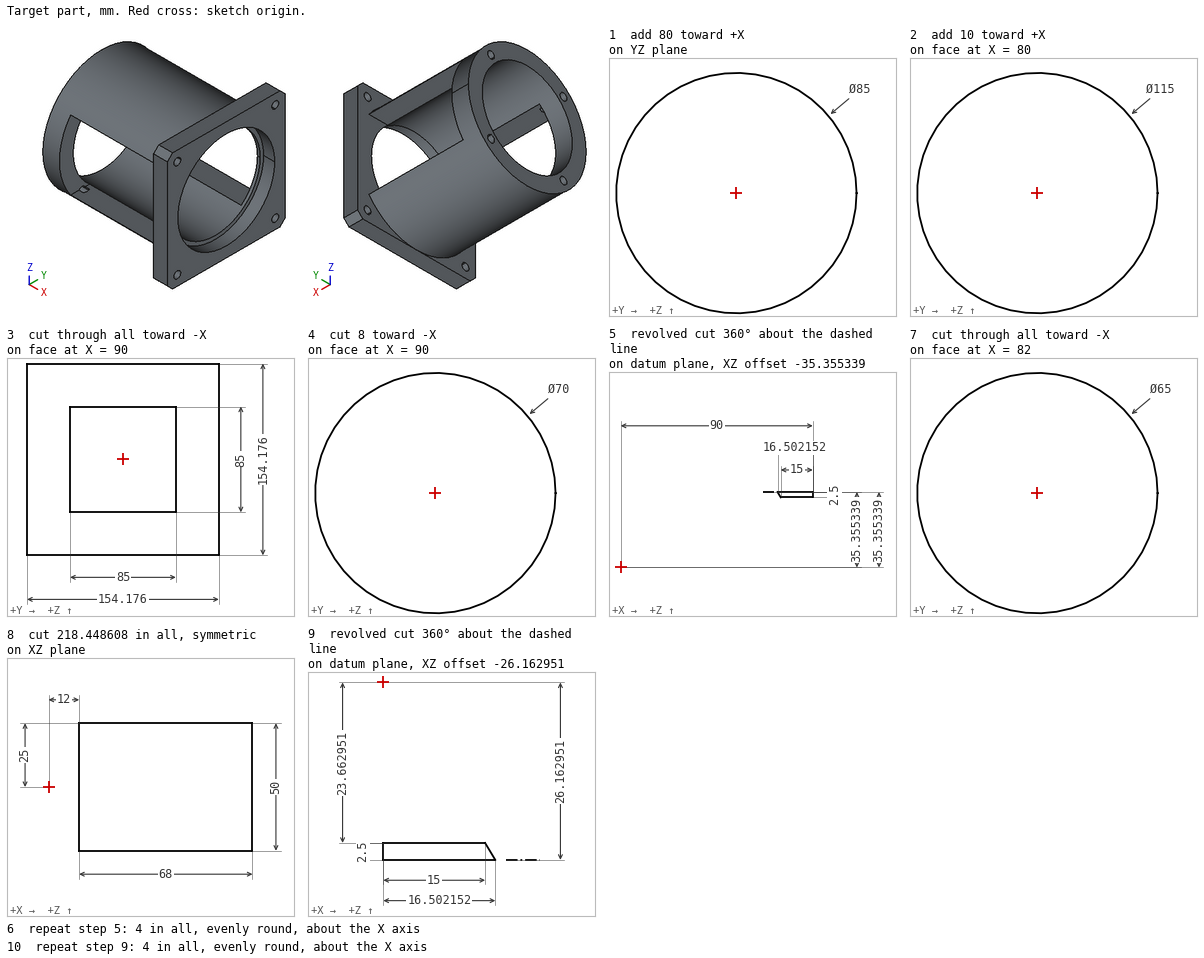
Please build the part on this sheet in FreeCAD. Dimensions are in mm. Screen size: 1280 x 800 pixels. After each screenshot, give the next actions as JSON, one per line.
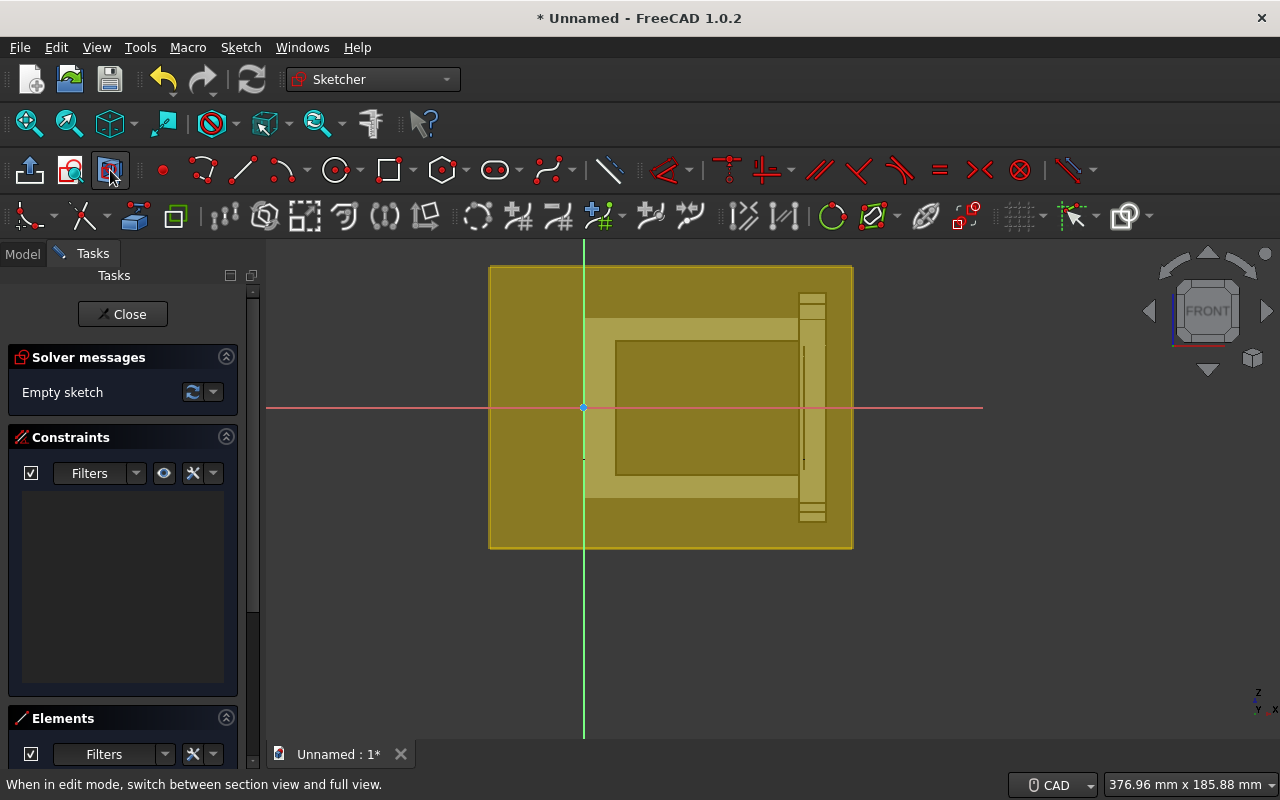
{"action": "scroll", "coordinate": [585, 428], "scroll_direction": "up", "scroll_amount": 7}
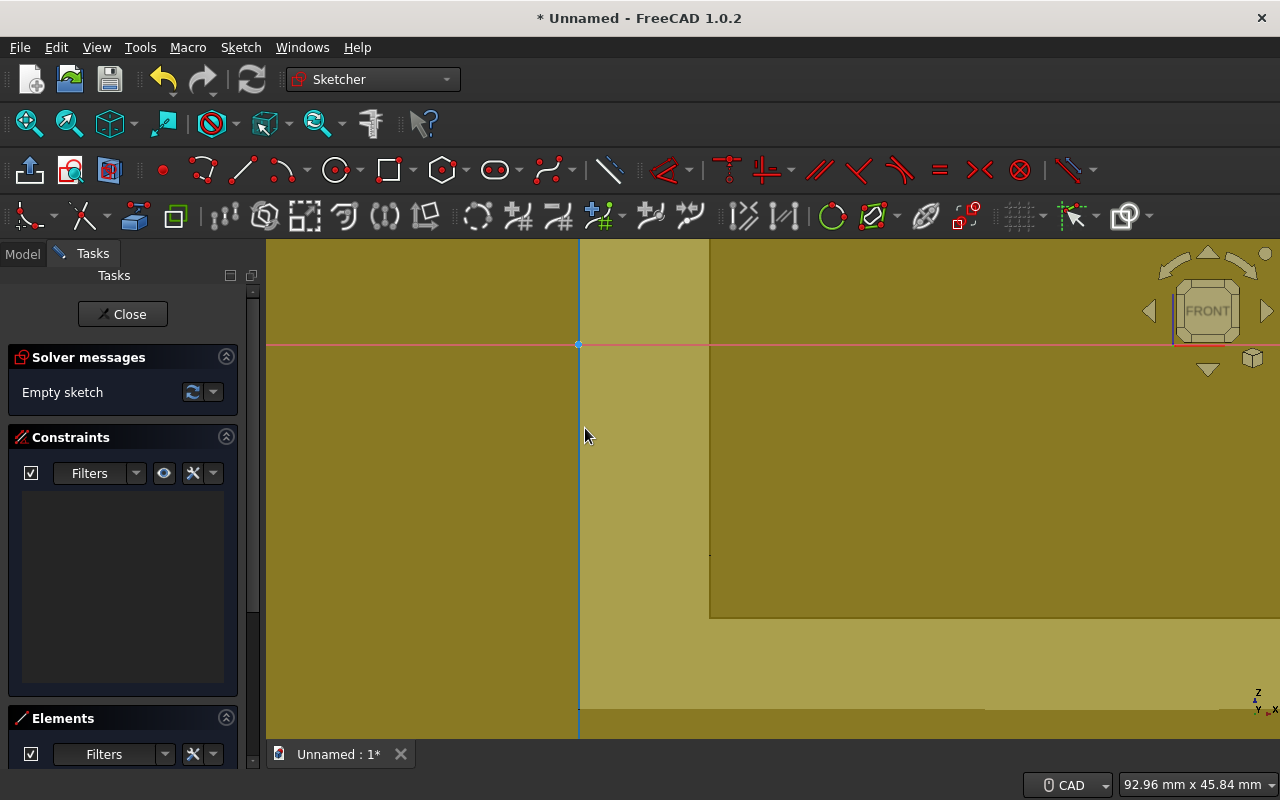
{"action": "left_click", "coordinate": [204, 170]}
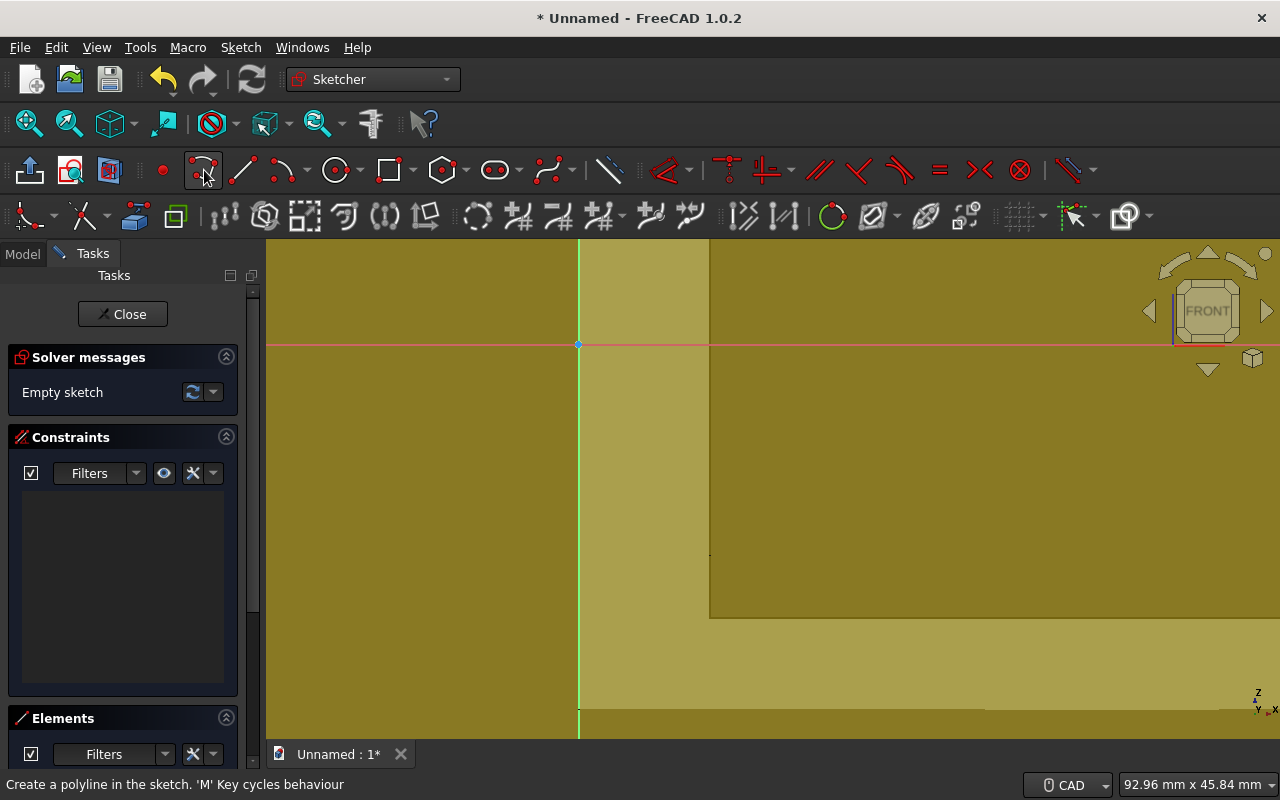
{"action": "left_click", "coordinate": [579, 603]}
{"action": "left_click", "coordinate": [742, 603]}
{"action": "left_click", "coordinate": [759, 630]}
{"action": "left_click", "coordinate": [588, 630]}
{"action": "left_click", "coordinate": [579, 604]}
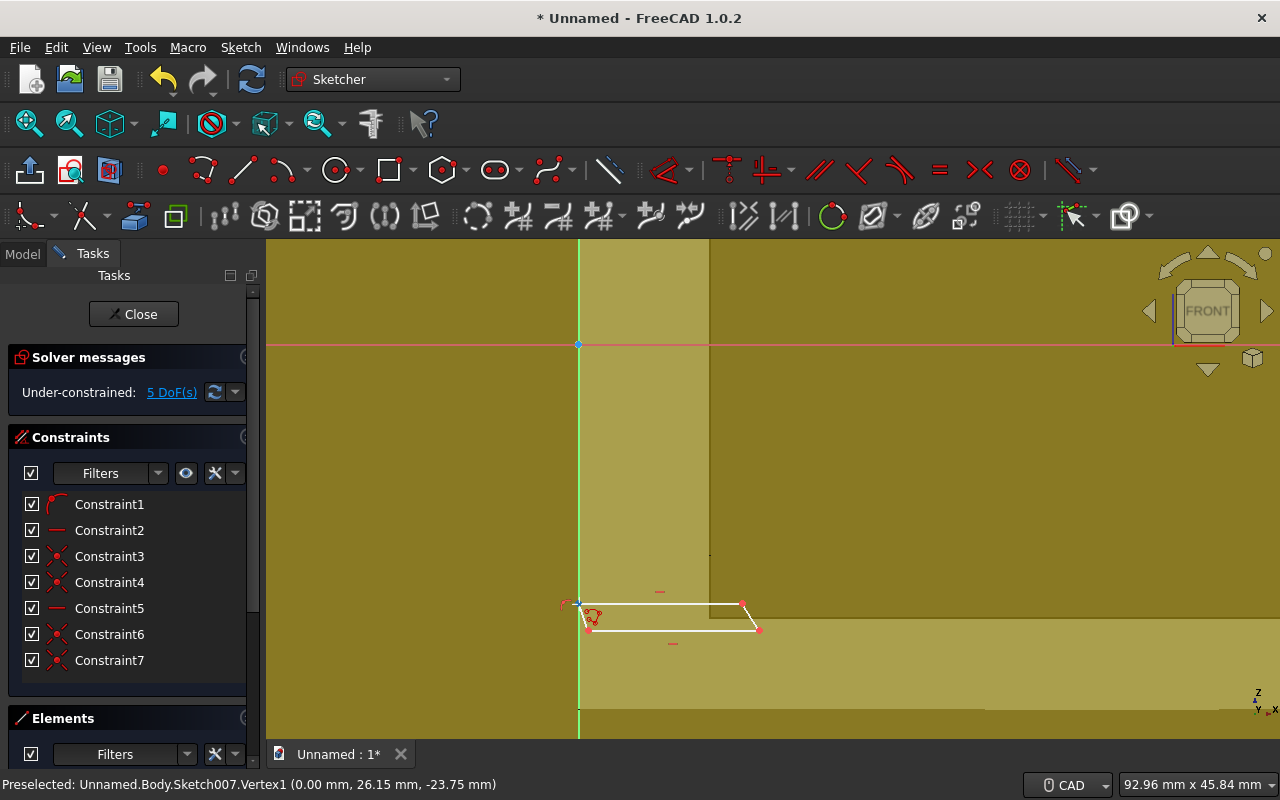
{"action": "left_click", "coordinate": [244, 170]}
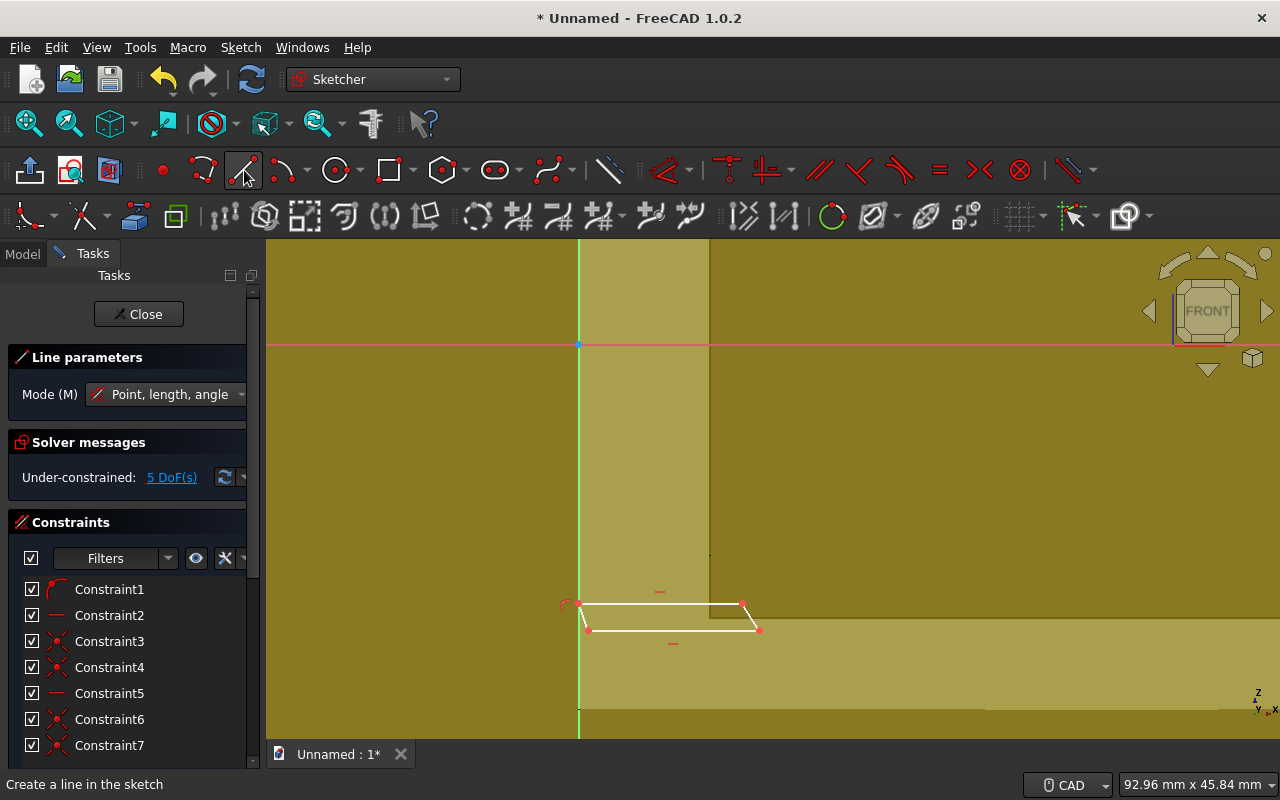
{"action": "left_click", "coordinate": [777, 630]}
{"action": "left_click", "coordinate": [831, 630]}
{"action": "key", "text": "Escape"}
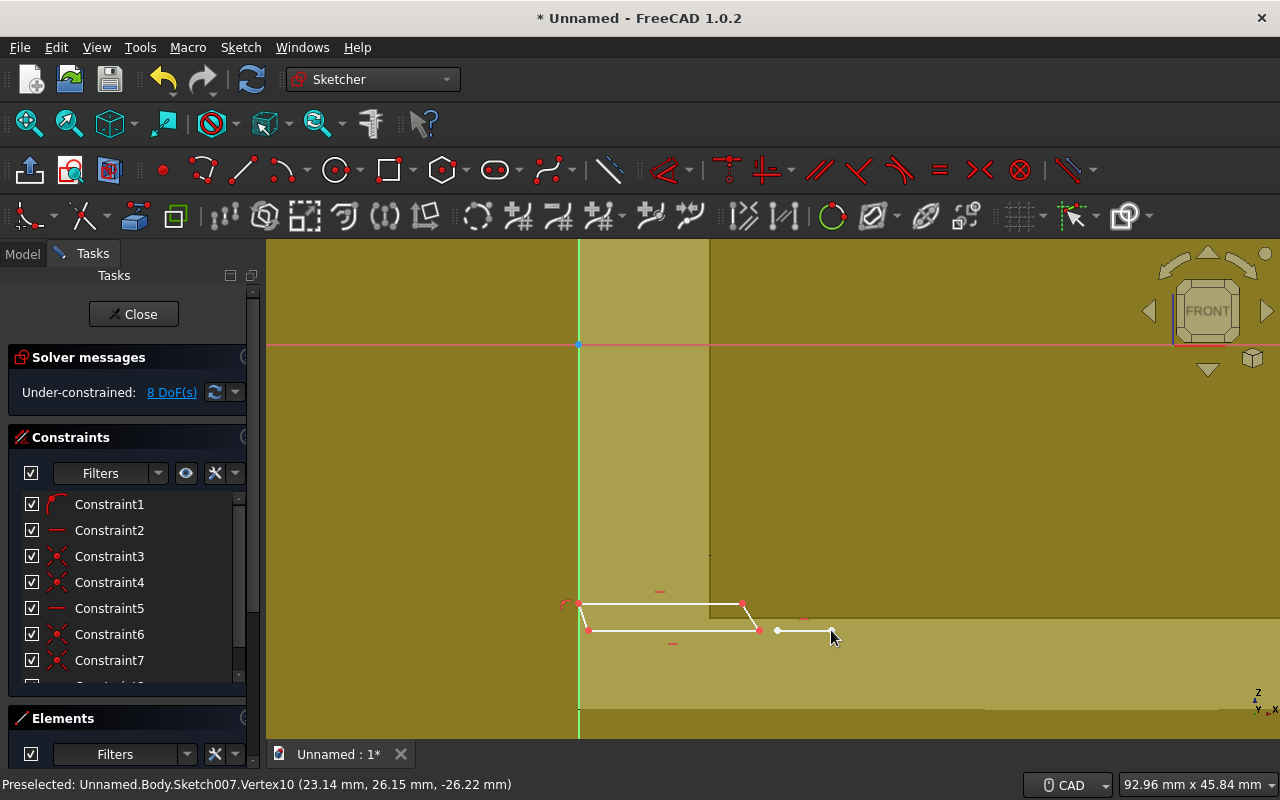
{"action": "left_click", "coordinate": [793, 631]}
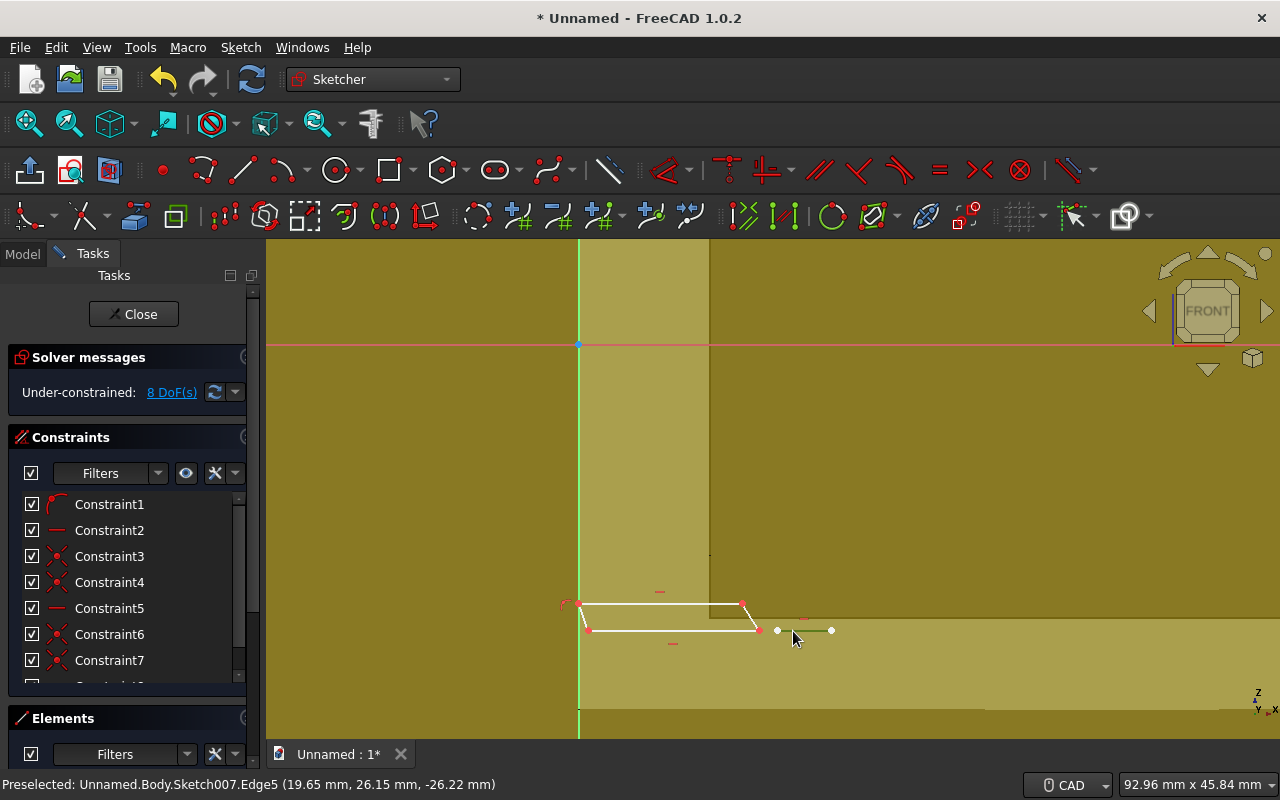
{"action": "key", "text": "g n"}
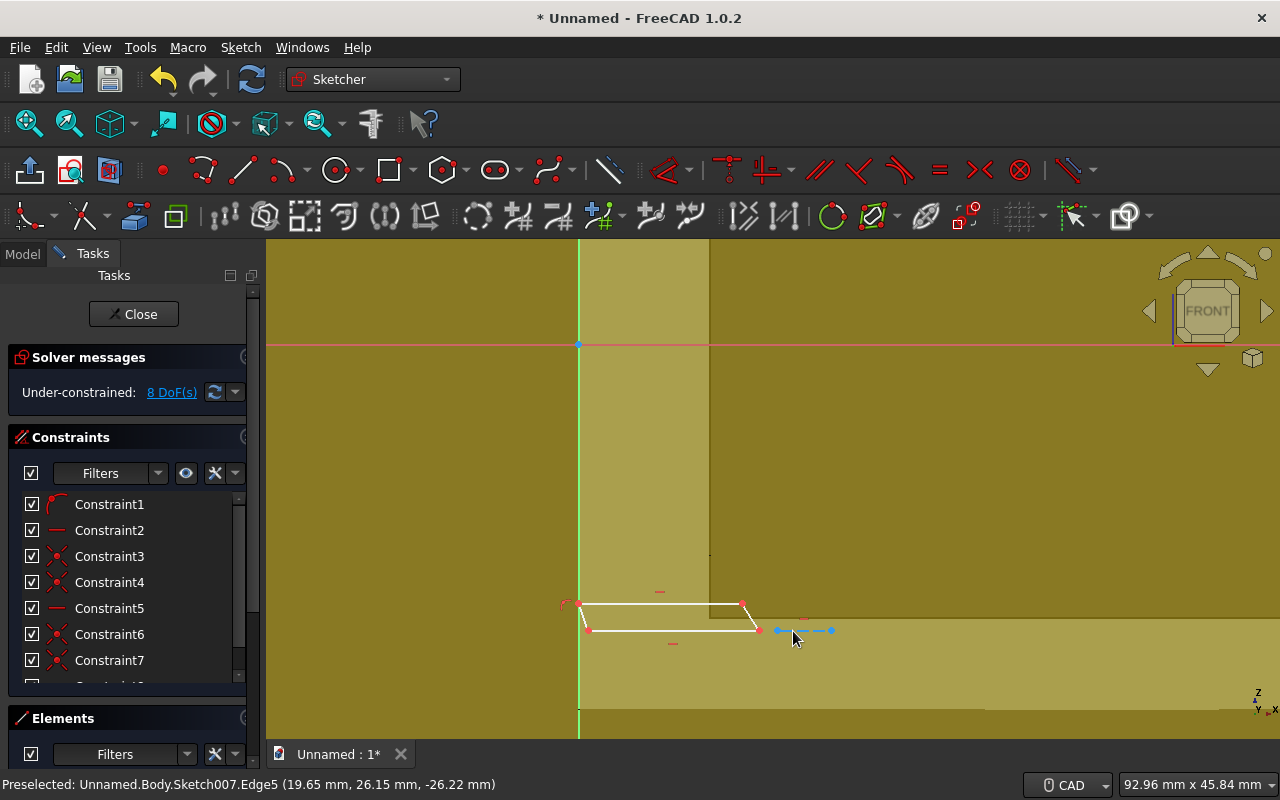
{"action": "scroll", "coordinate": [582, 615], "scroll_direction": "up", "scroll_amount": 2}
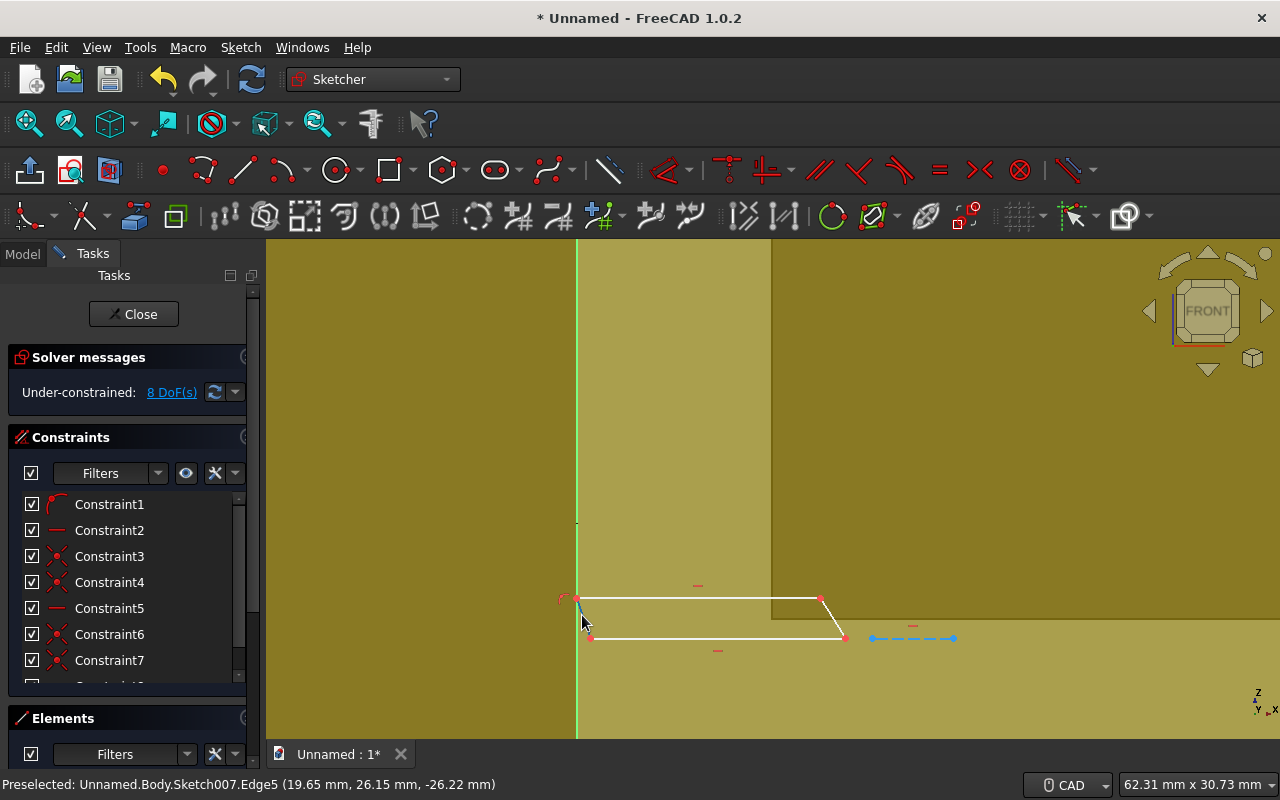
{"action": "left_click", "coordinate": [582, 614]}